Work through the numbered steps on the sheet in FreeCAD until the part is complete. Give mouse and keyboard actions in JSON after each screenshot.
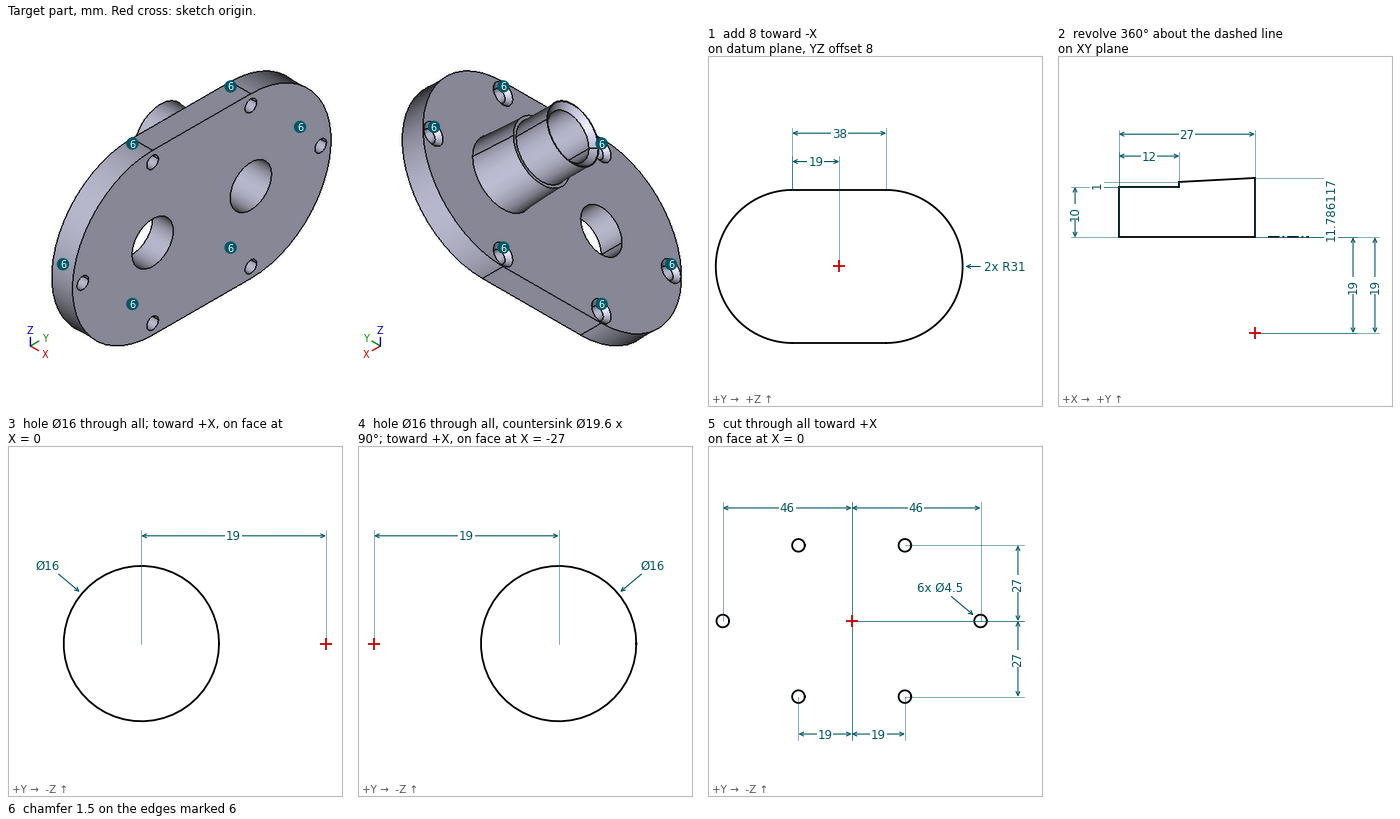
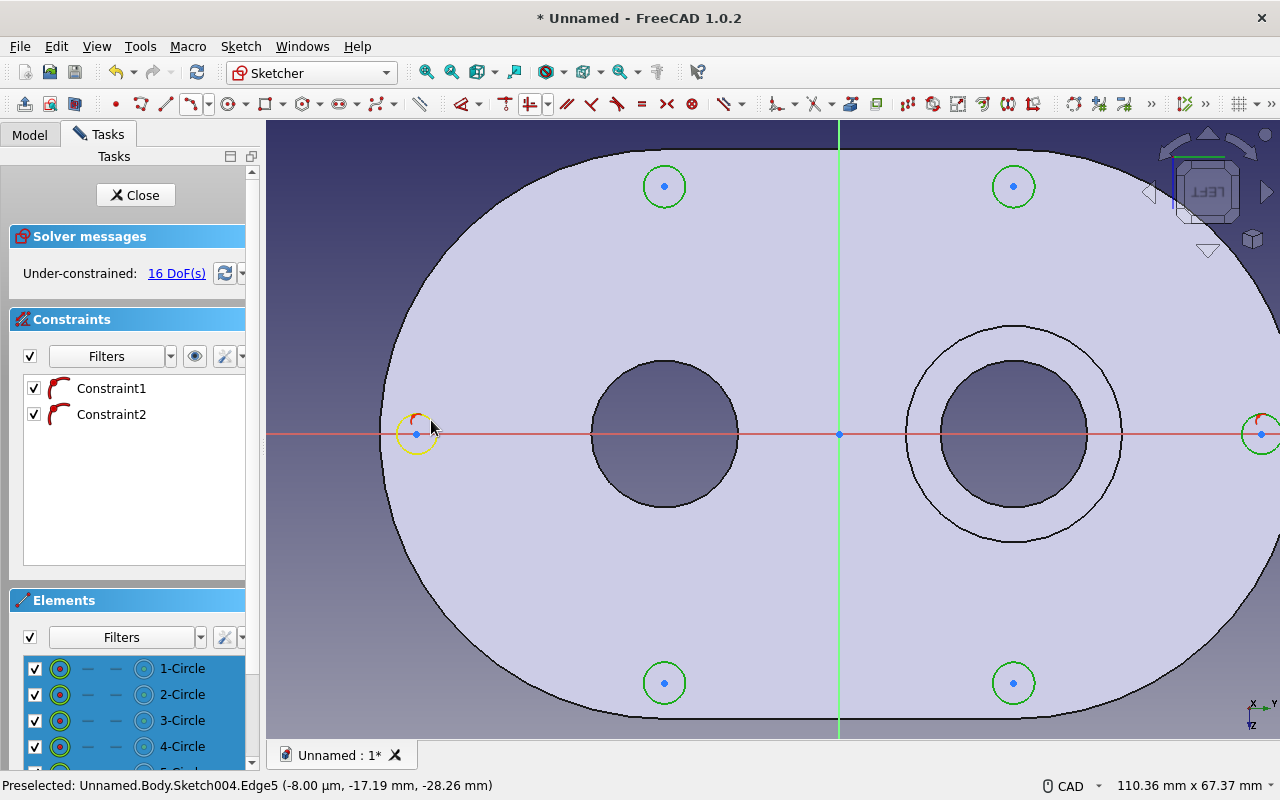
{"action": "left_click", "coordinate": [431, 420]}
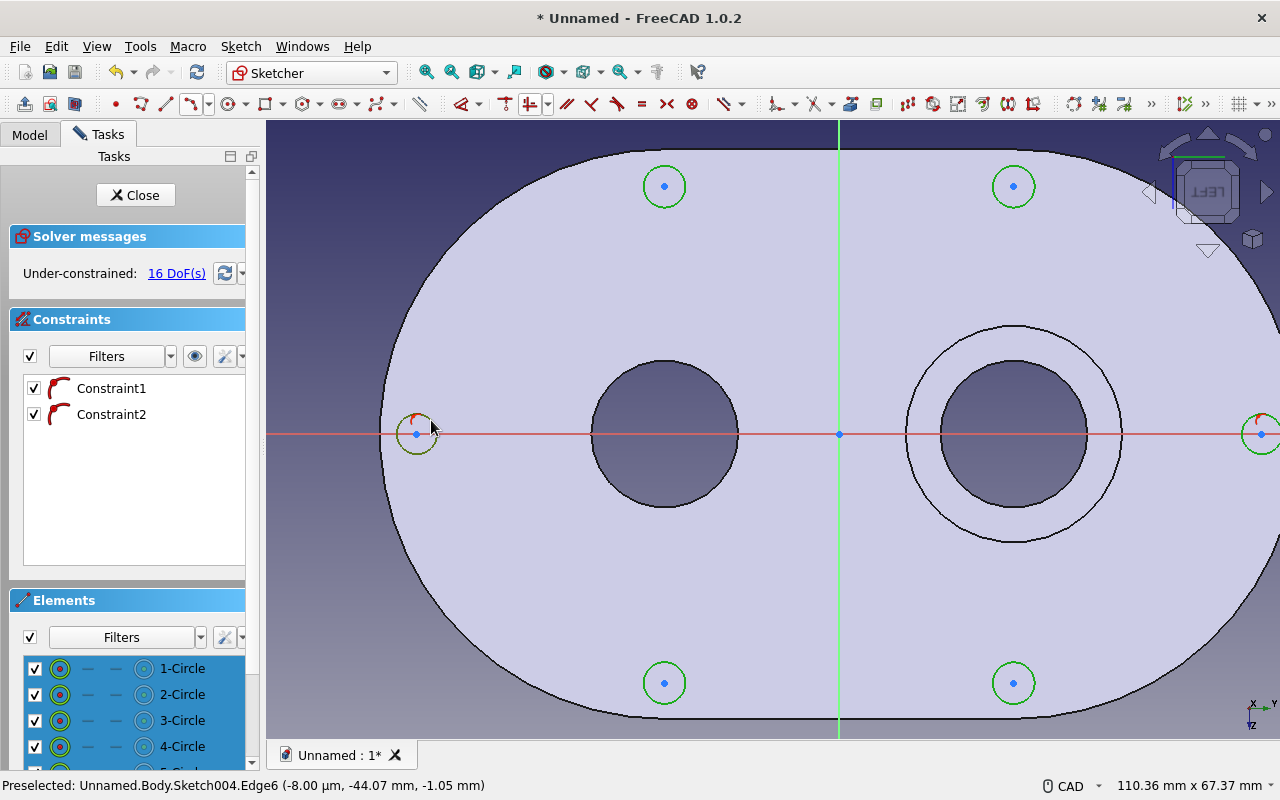
{"action": "key", "text": "e"}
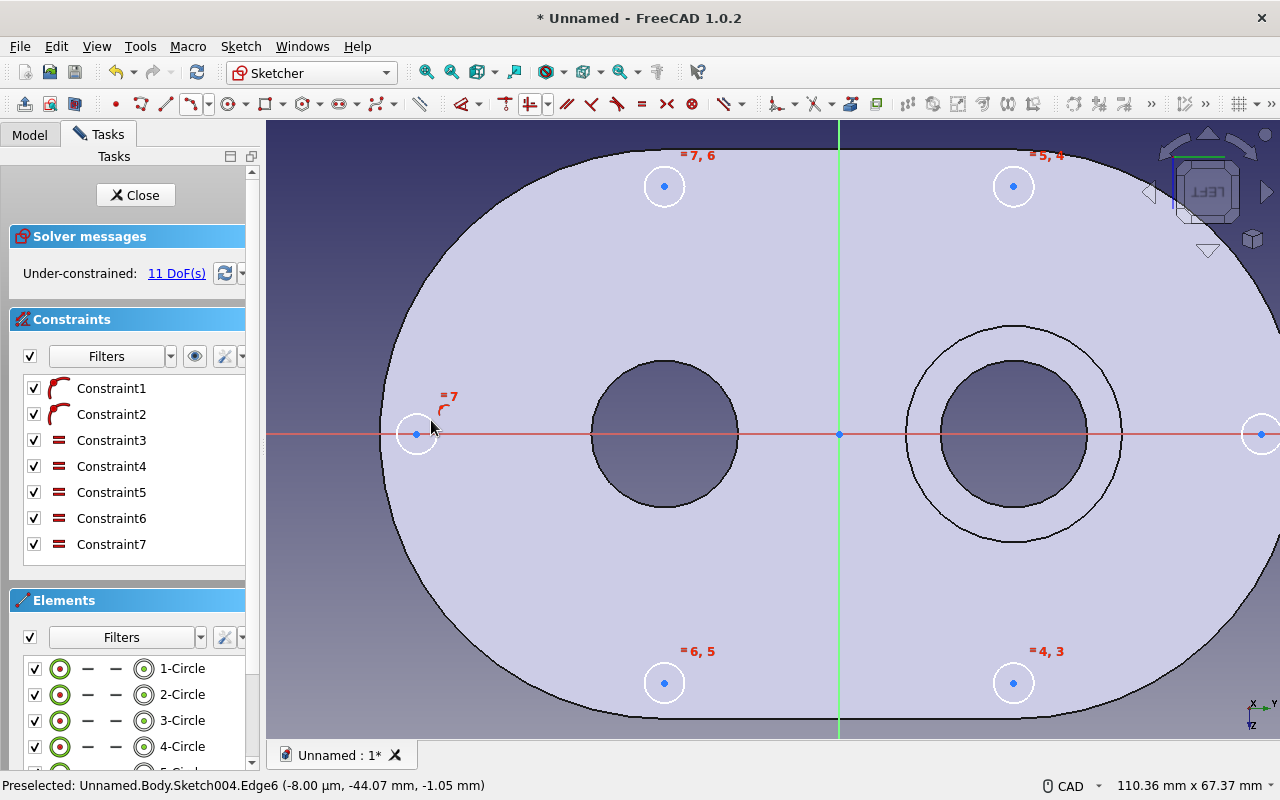
{"action": "left_click", "coordinate": [1014, 683]}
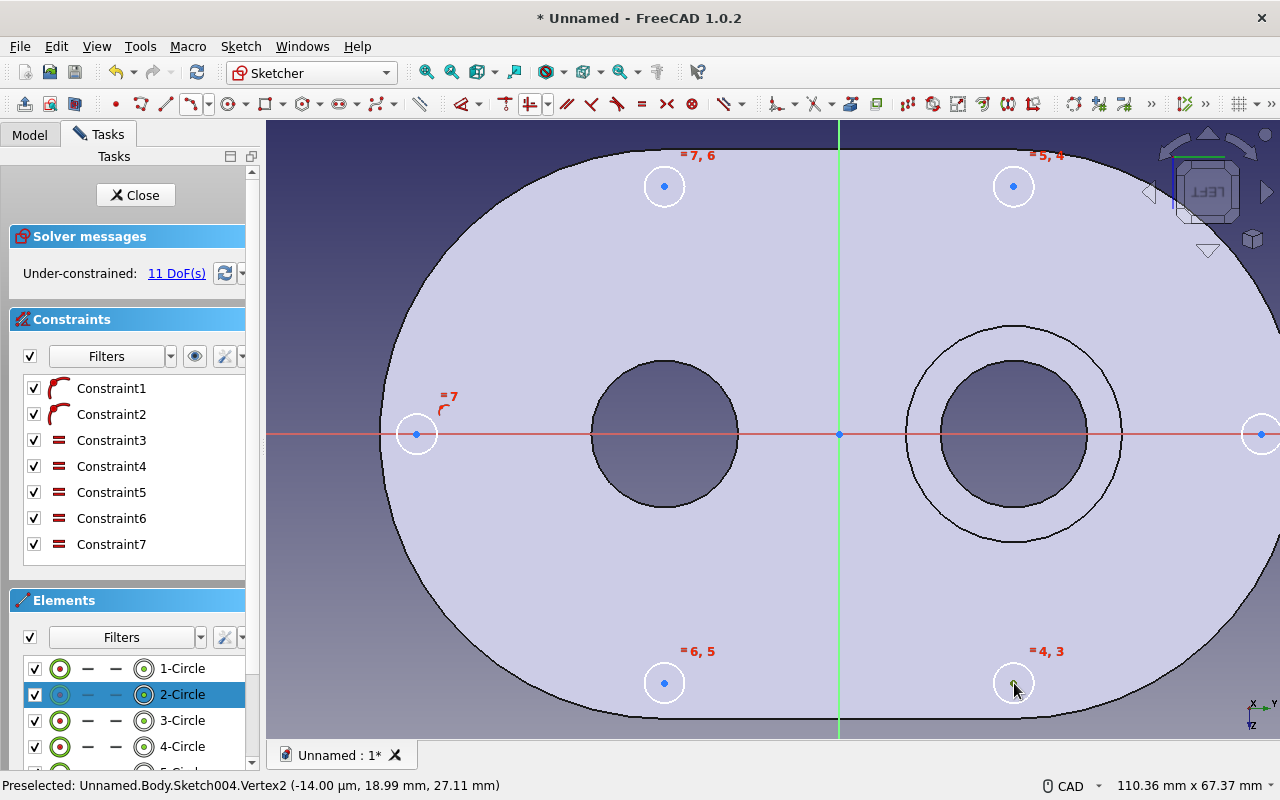
{"action": "left_click", "coordinate": [1014, 187]}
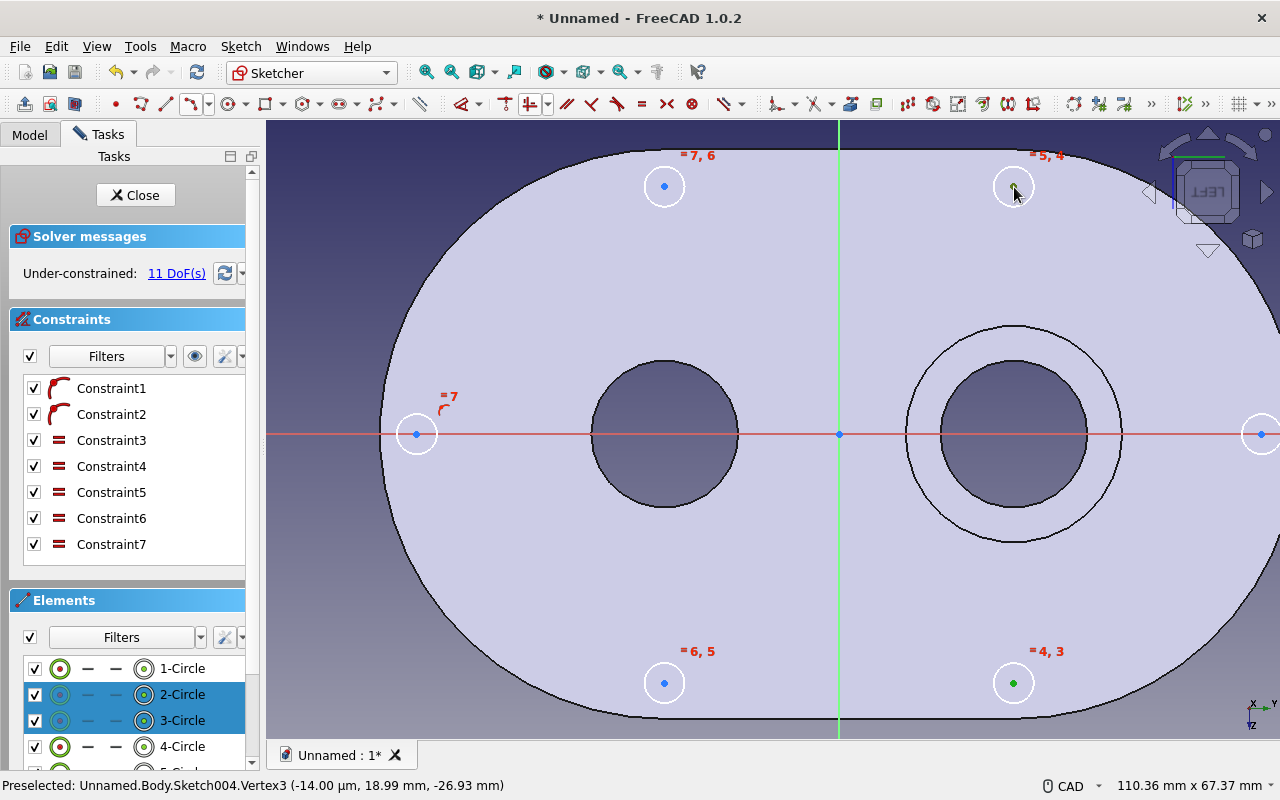
{"action": "left_click", "coordinate": [548, 104]}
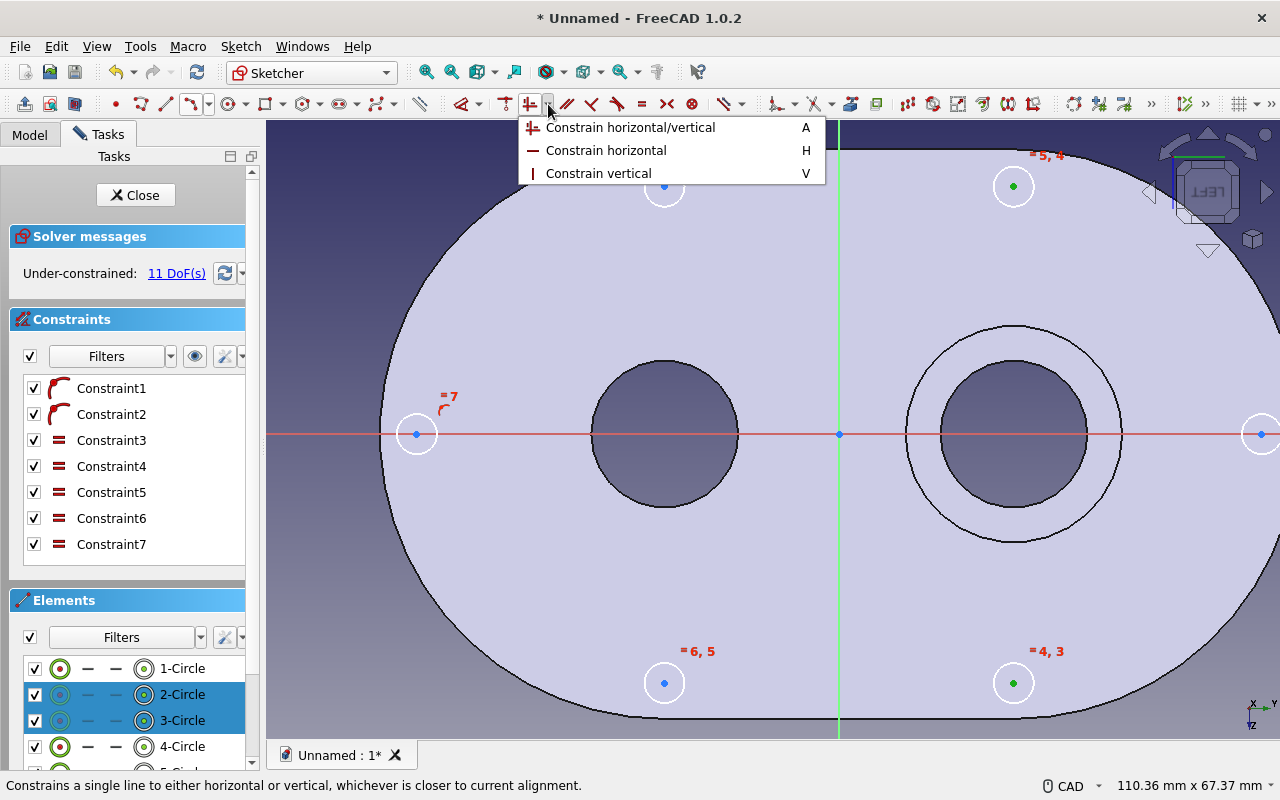
{"action": "left_click", "coordinate": [672, 174]}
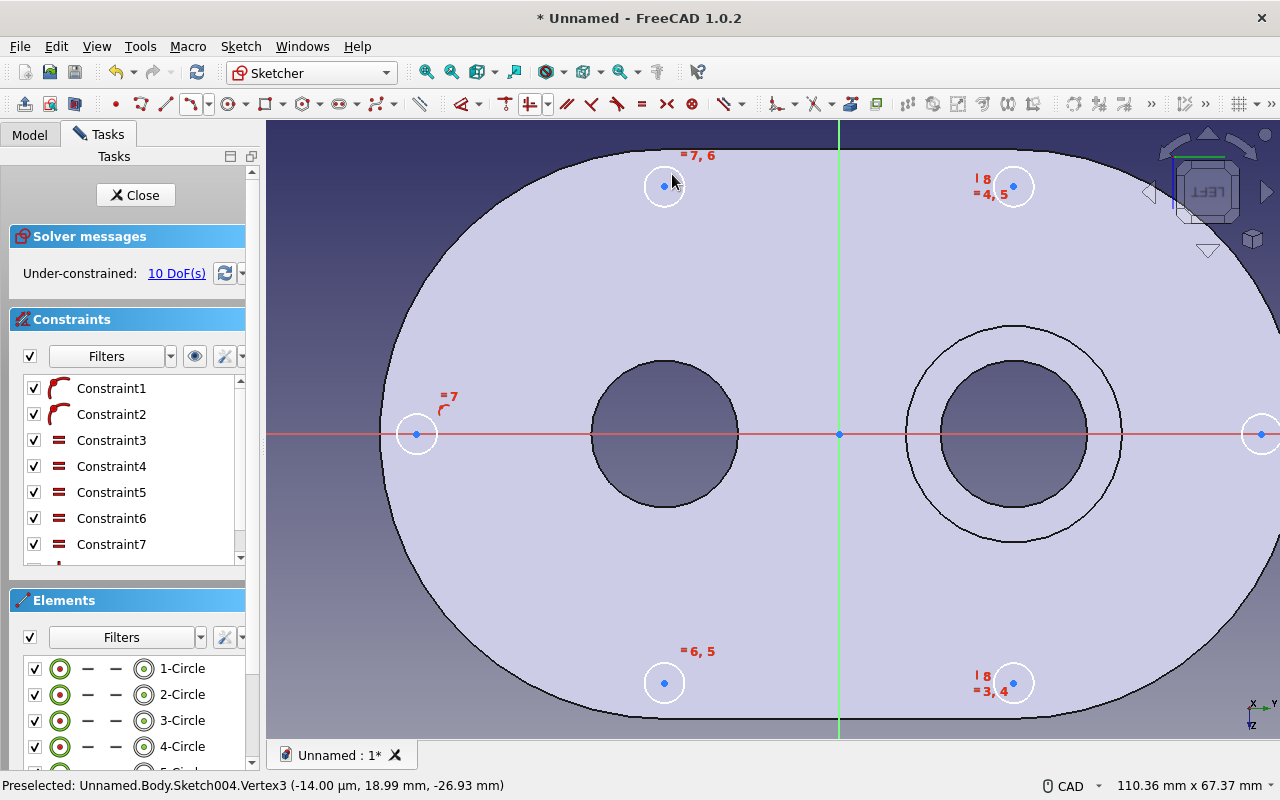
{"action": "left_click", "coordinate": [1014, 683]}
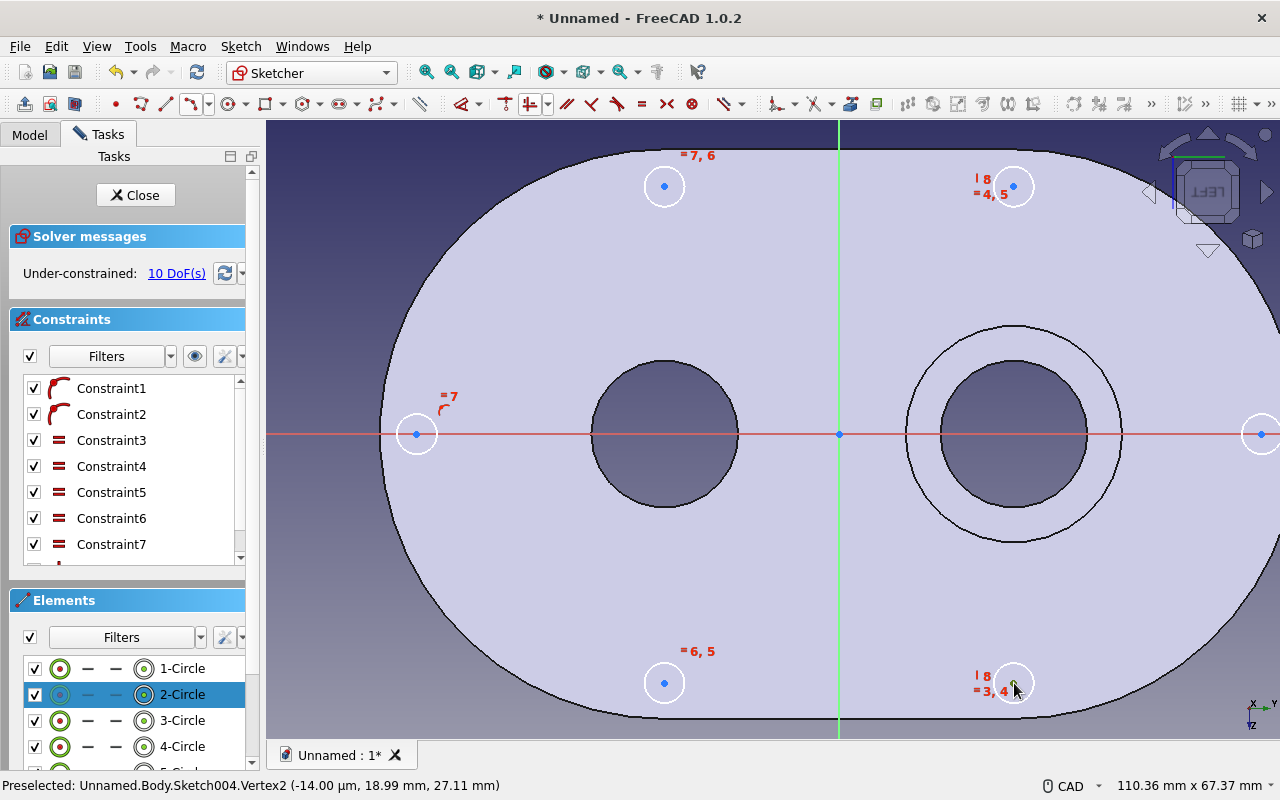
{"action": "left_click", "coordinate": [665, 683]}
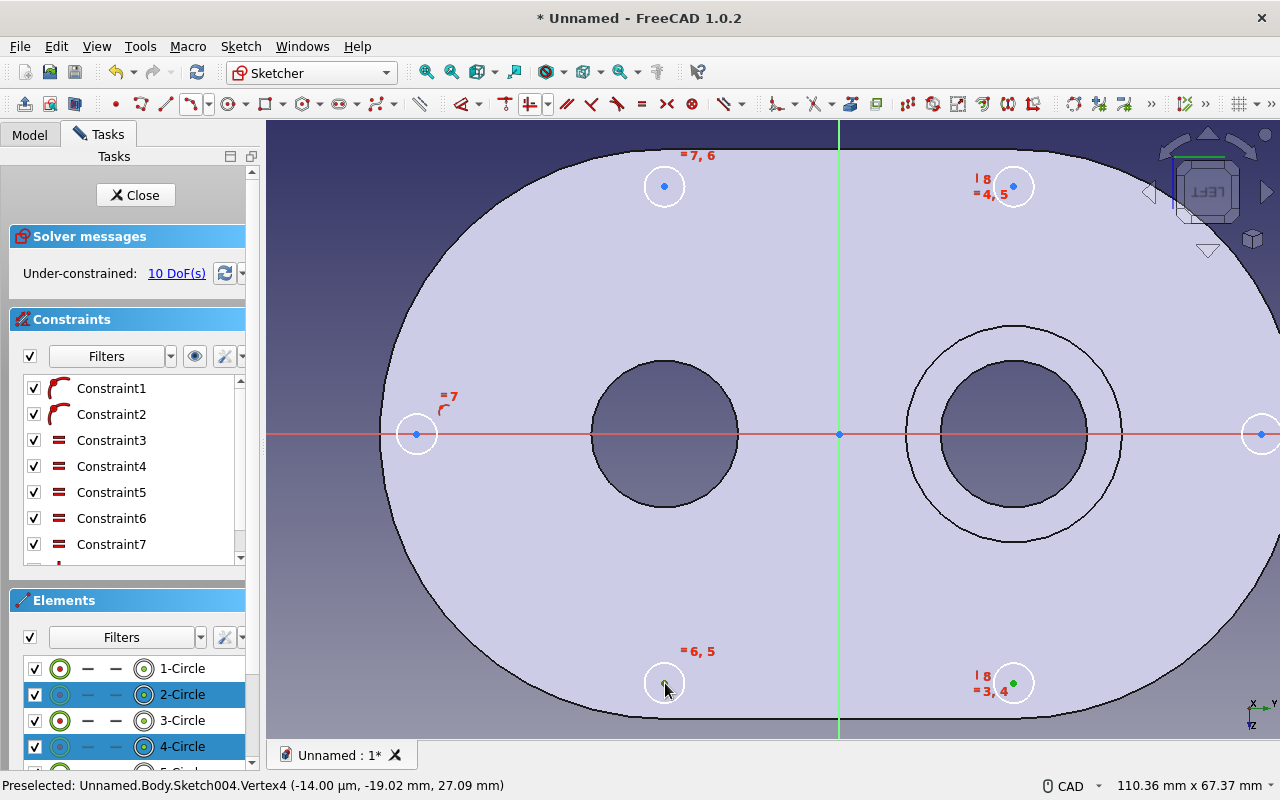
{"action": "key", "text": "h"}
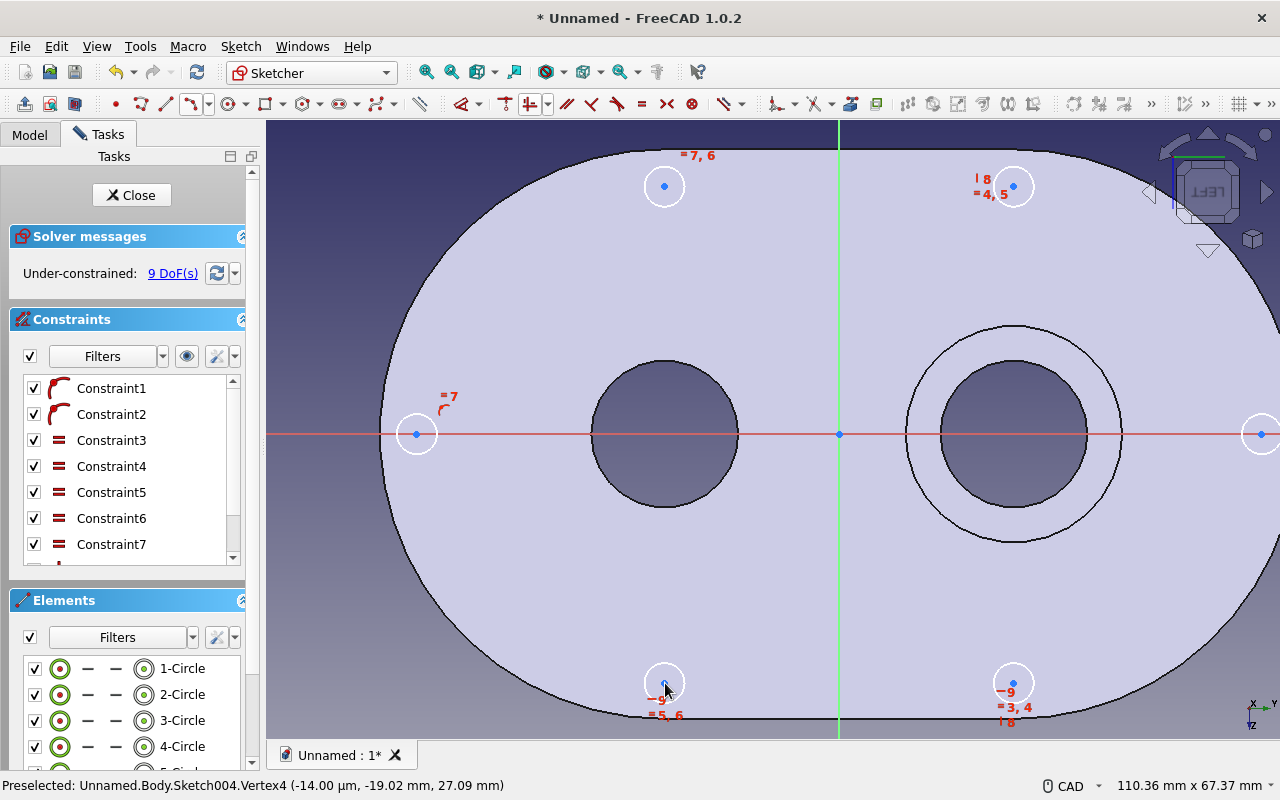
{"action": "left_click", "coordinate": [665, 683]}